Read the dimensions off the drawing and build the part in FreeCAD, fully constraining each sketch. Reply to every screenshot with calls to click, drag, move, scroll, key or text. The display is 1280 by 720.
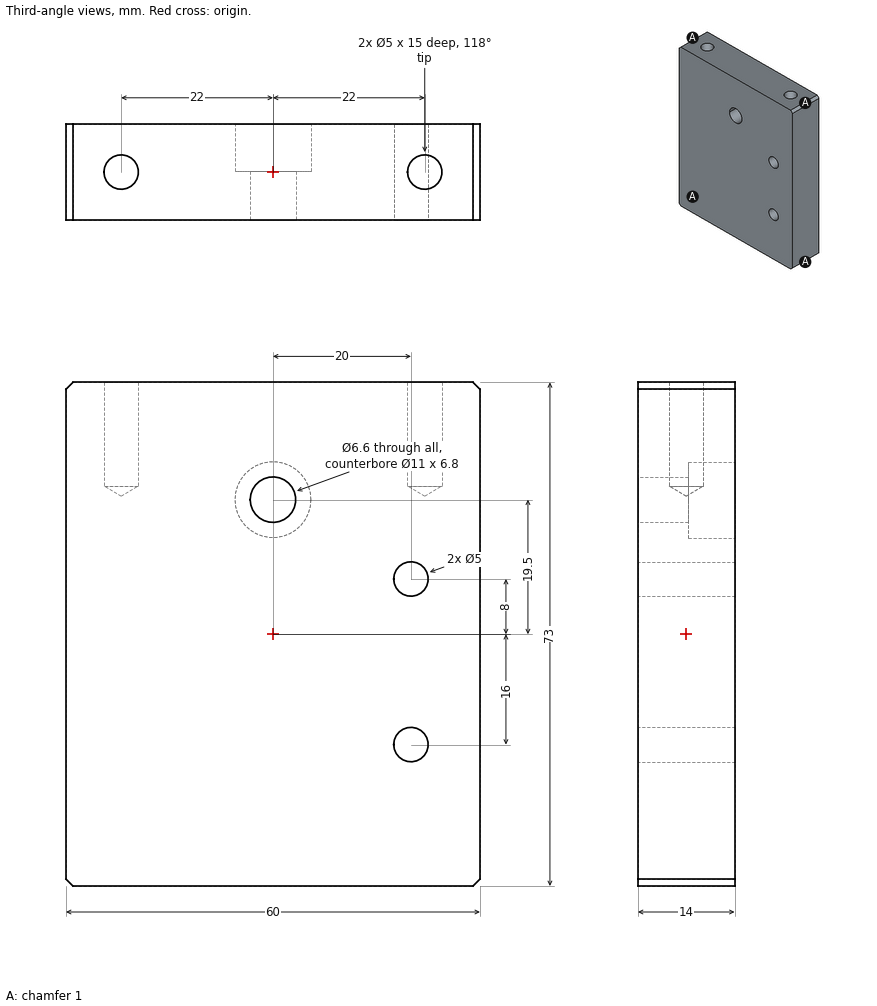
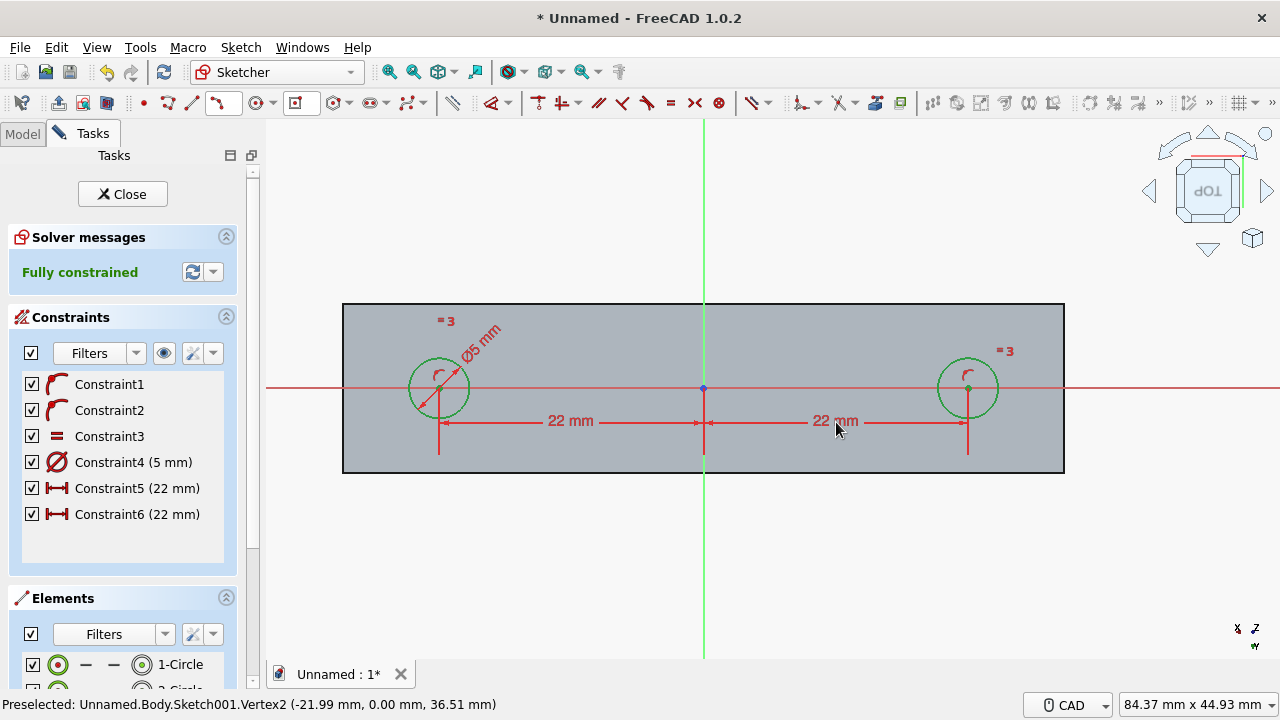
click(123, 194)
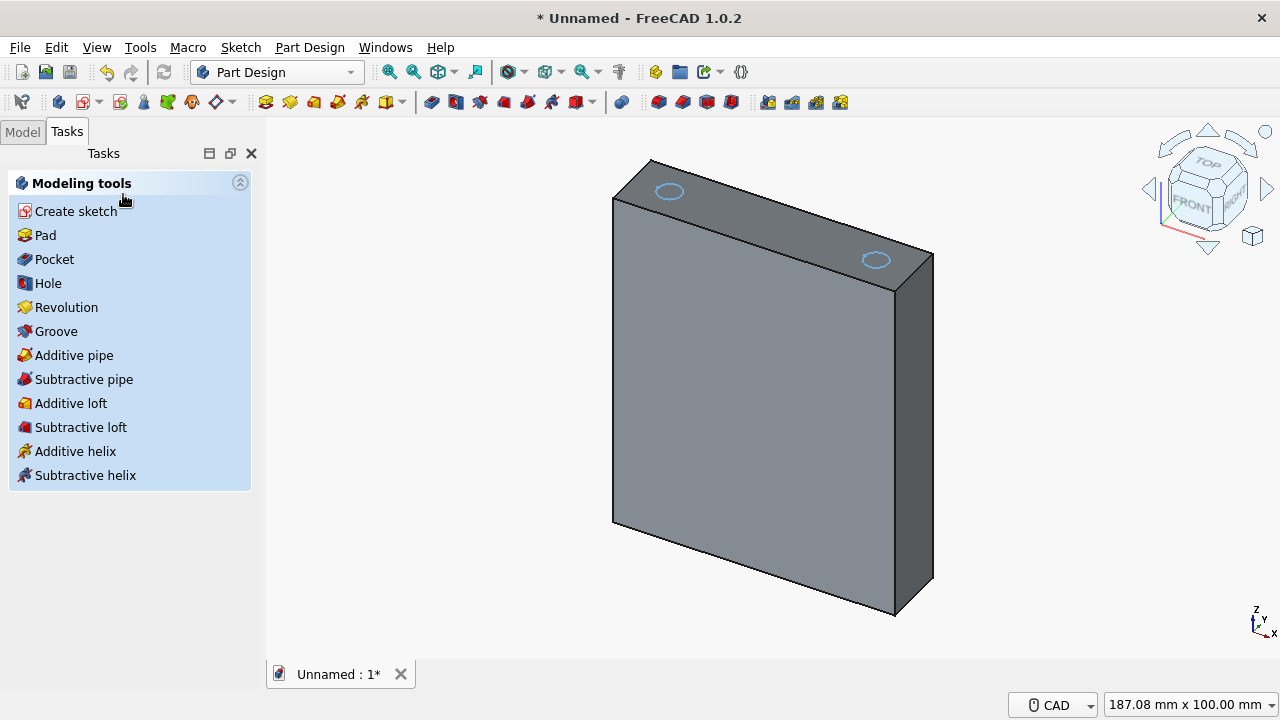
click(456, 102)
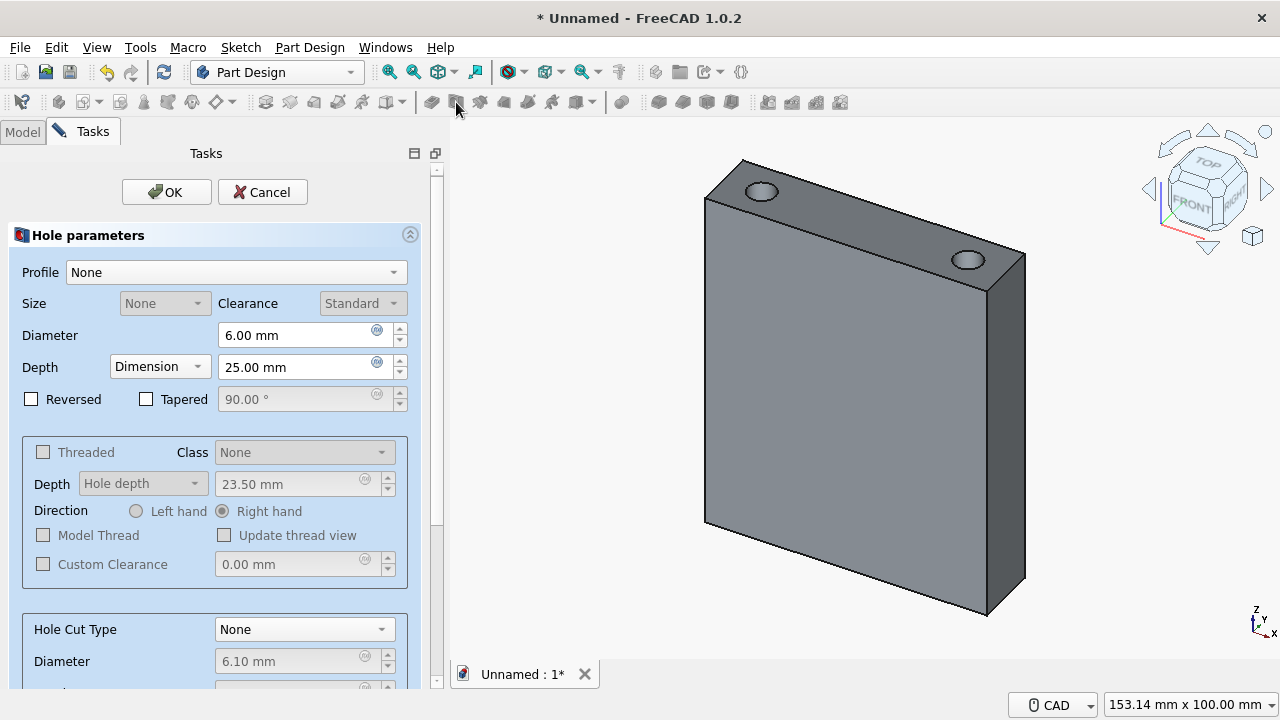
triple_click(305, 335)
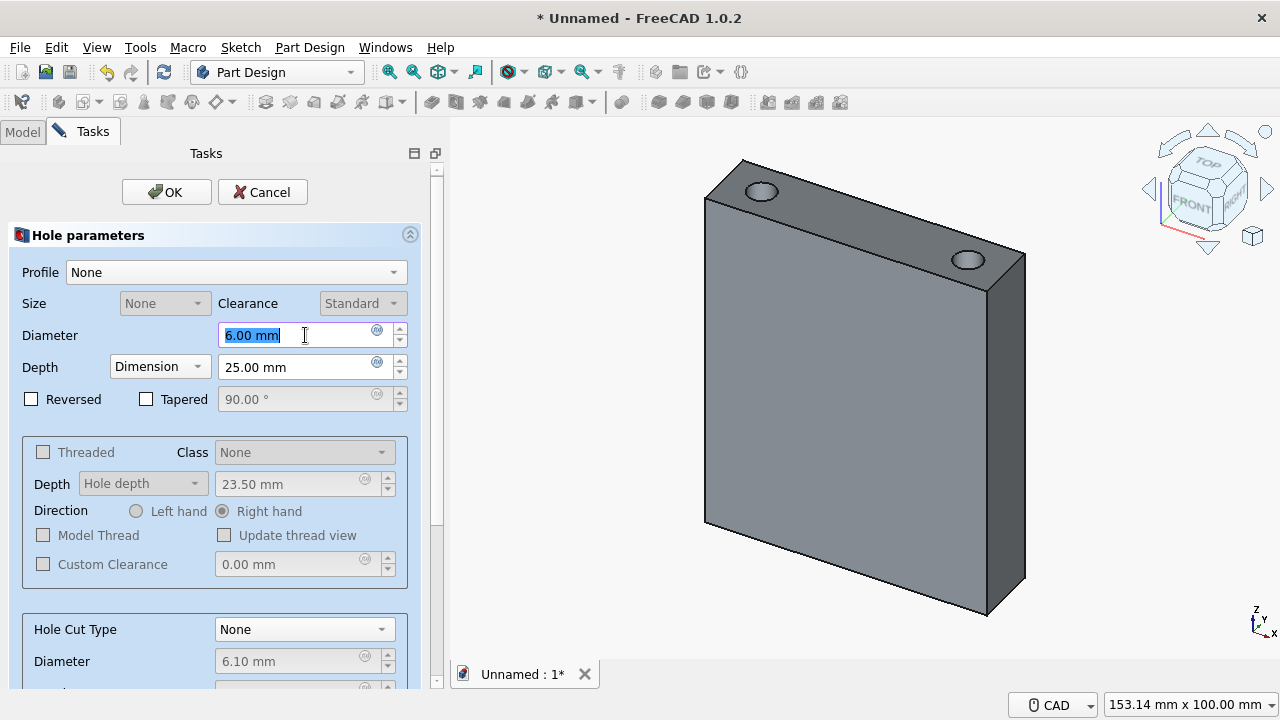
text(5)
key(Tab)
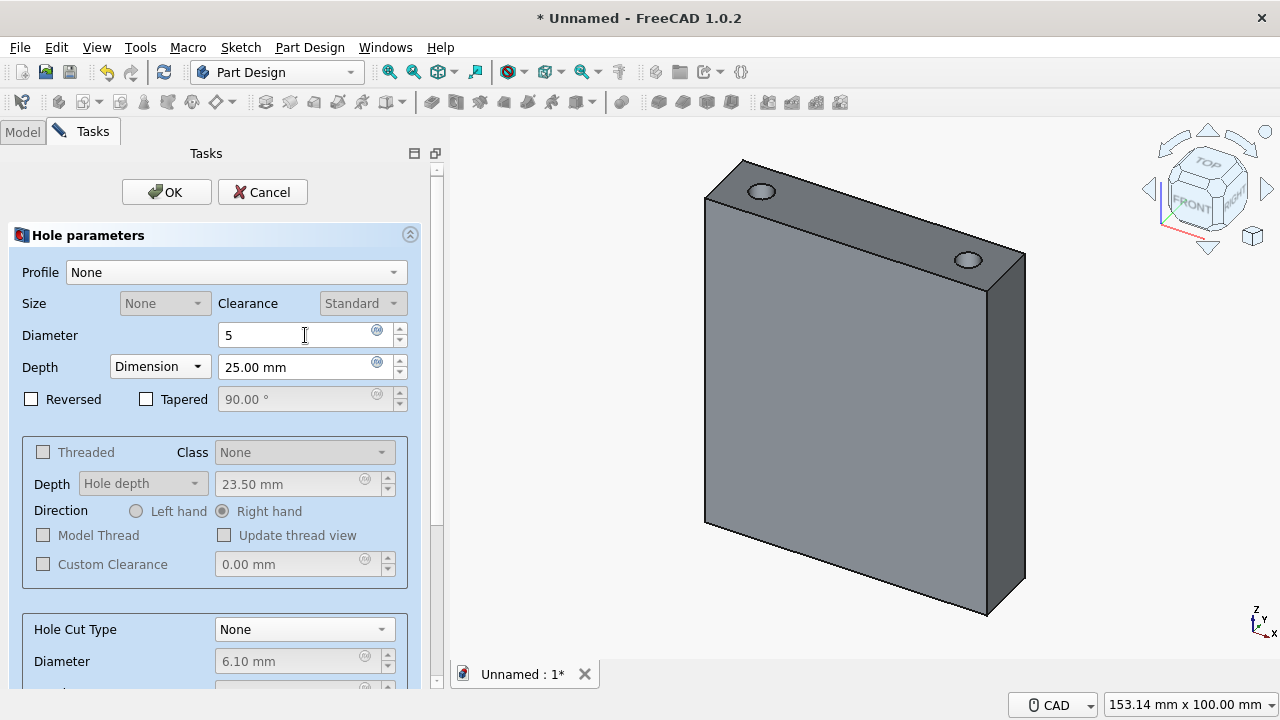
triple_click(305, 367)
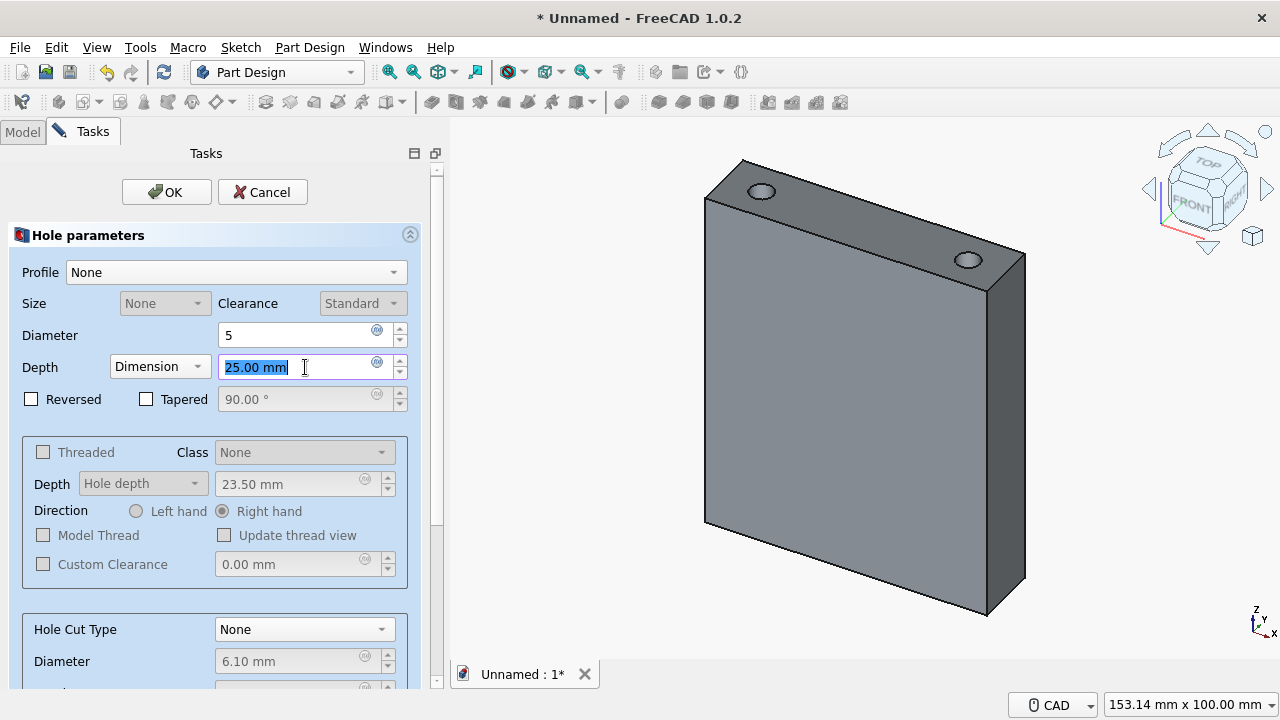
text(15)
key(Tab)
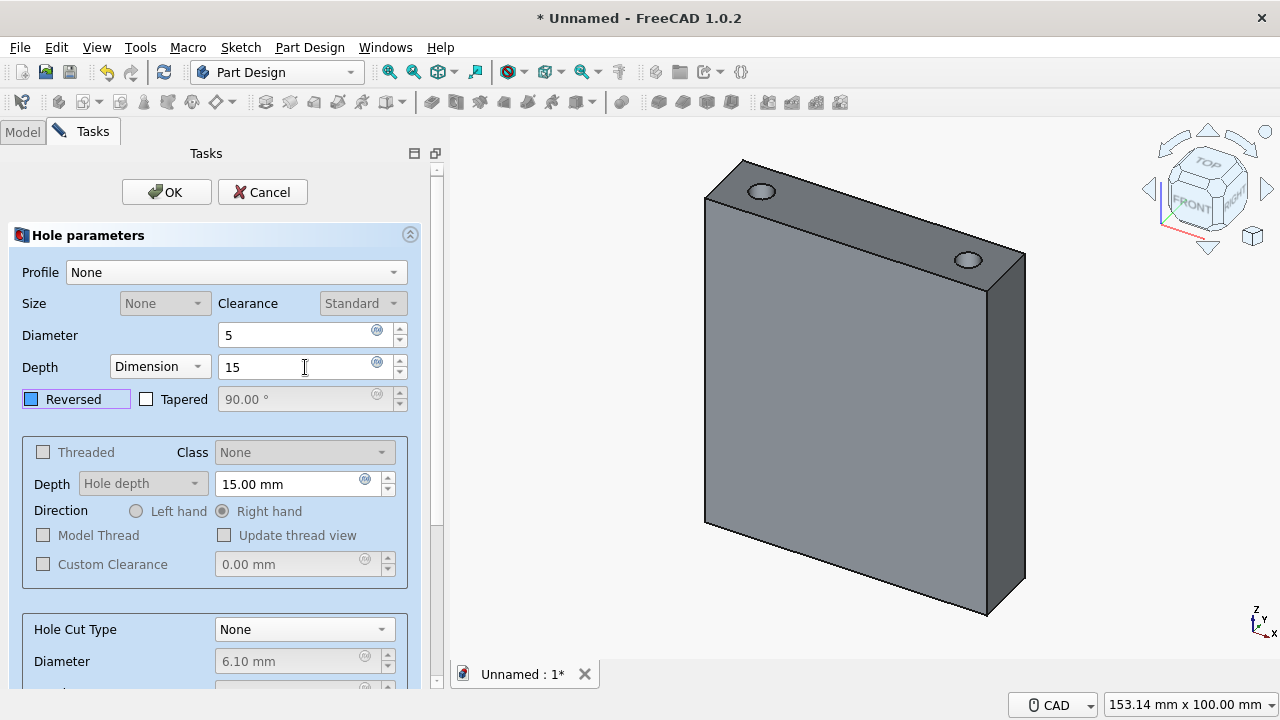
click(167, 192)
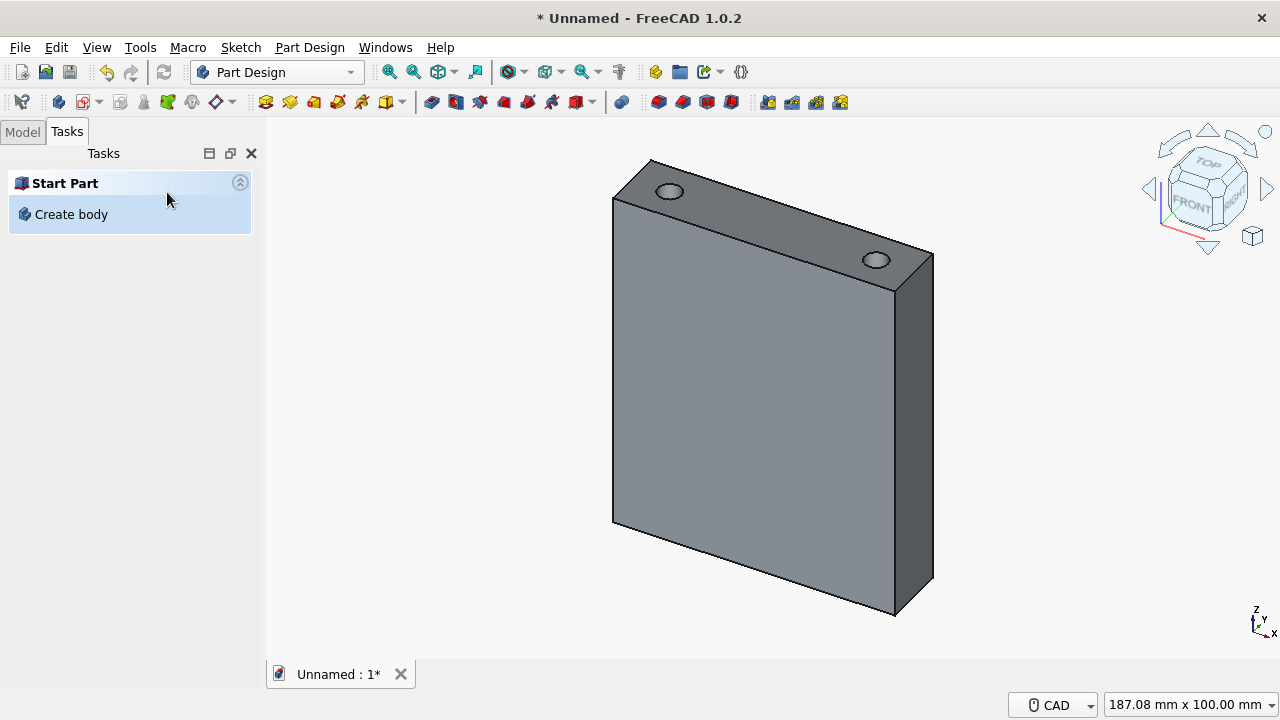
key(4)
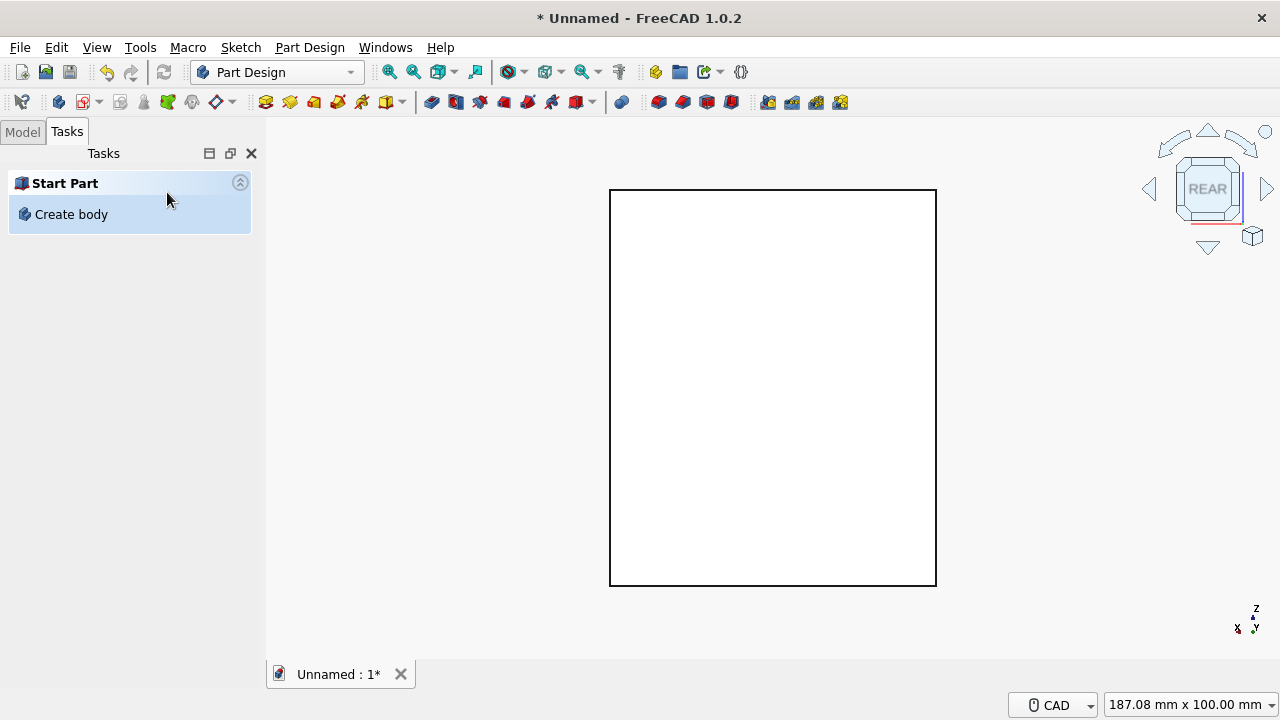
click(773, 387)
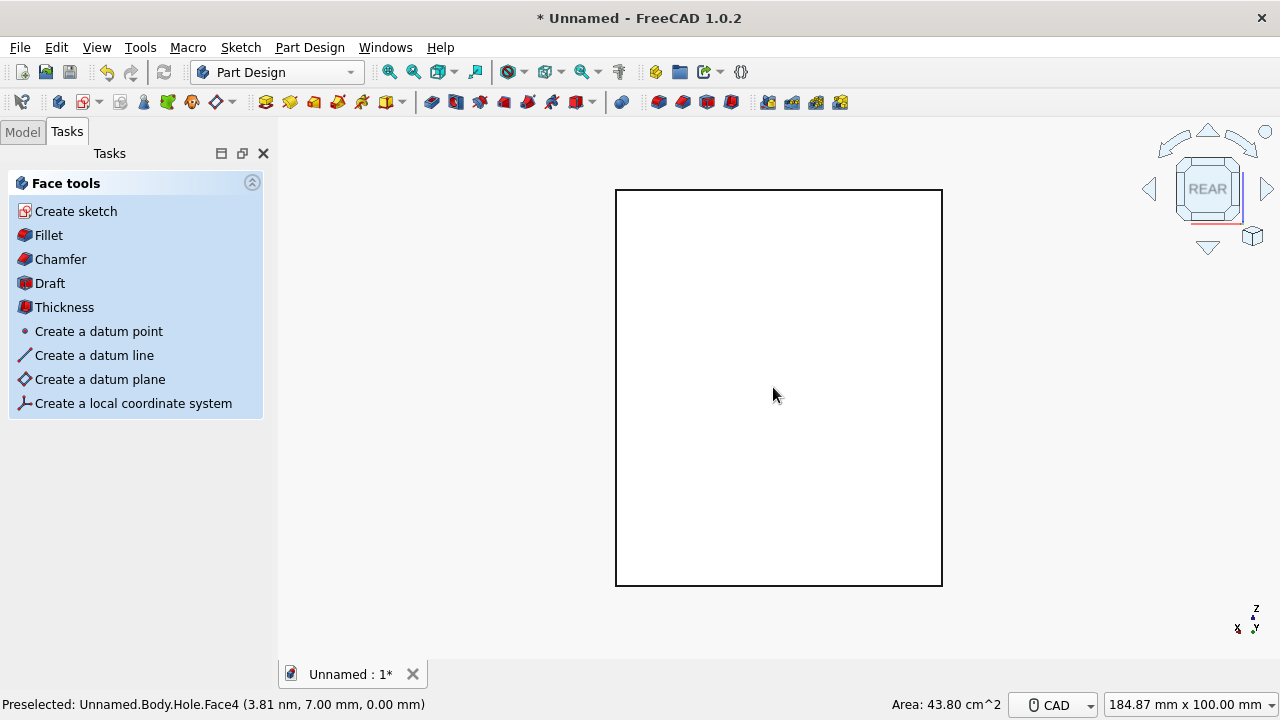
click(84, 102)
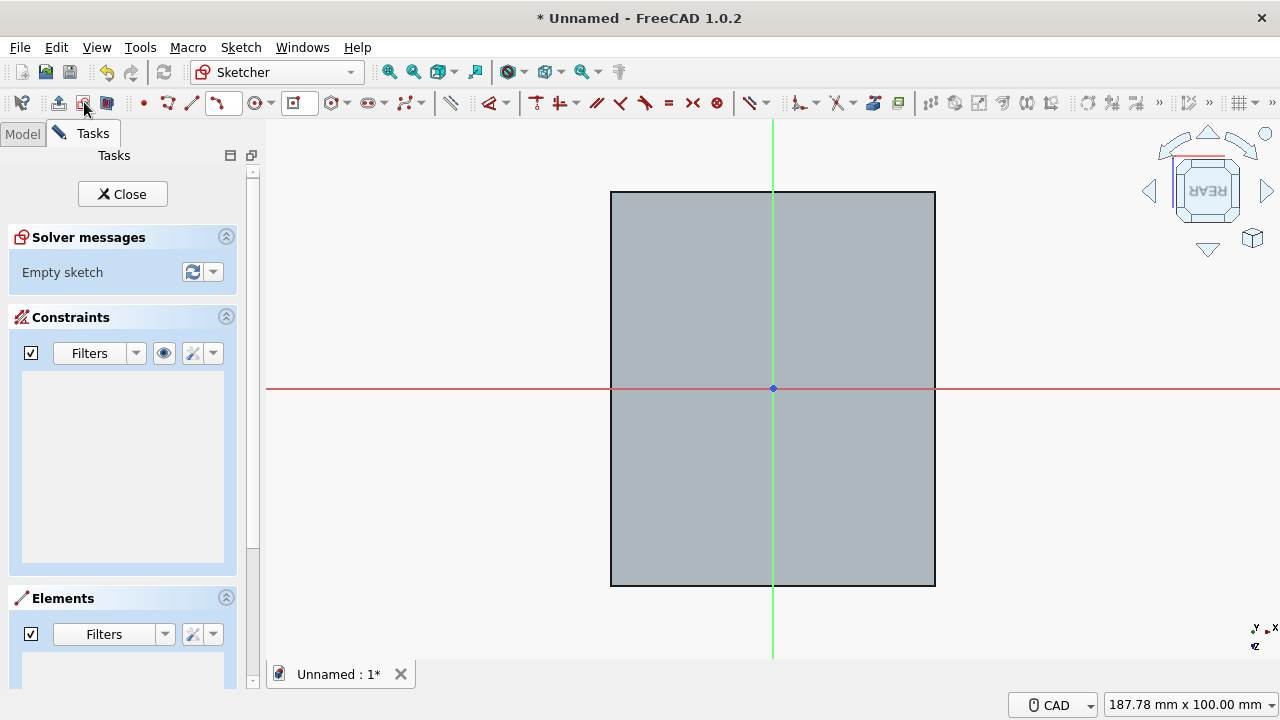
scroll(939, 350, up, 4)